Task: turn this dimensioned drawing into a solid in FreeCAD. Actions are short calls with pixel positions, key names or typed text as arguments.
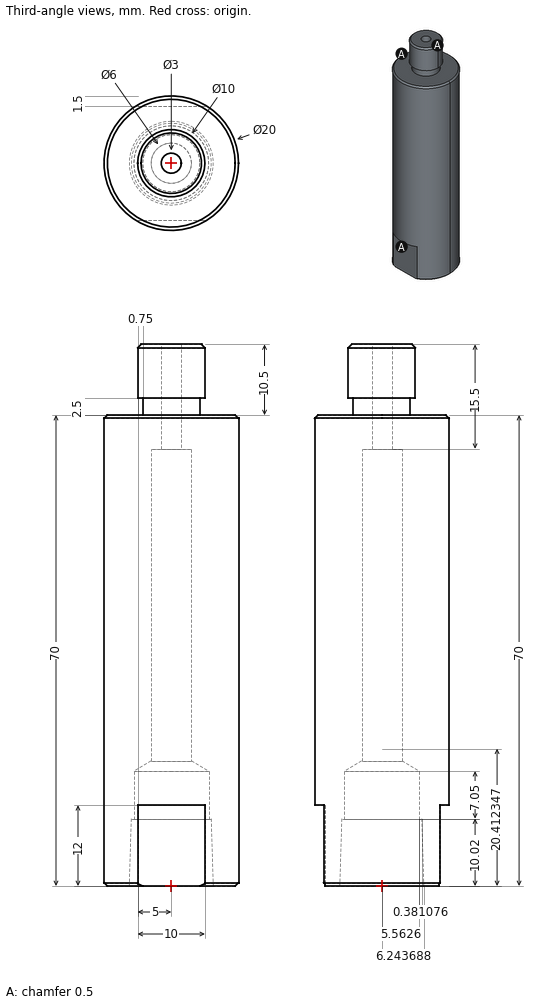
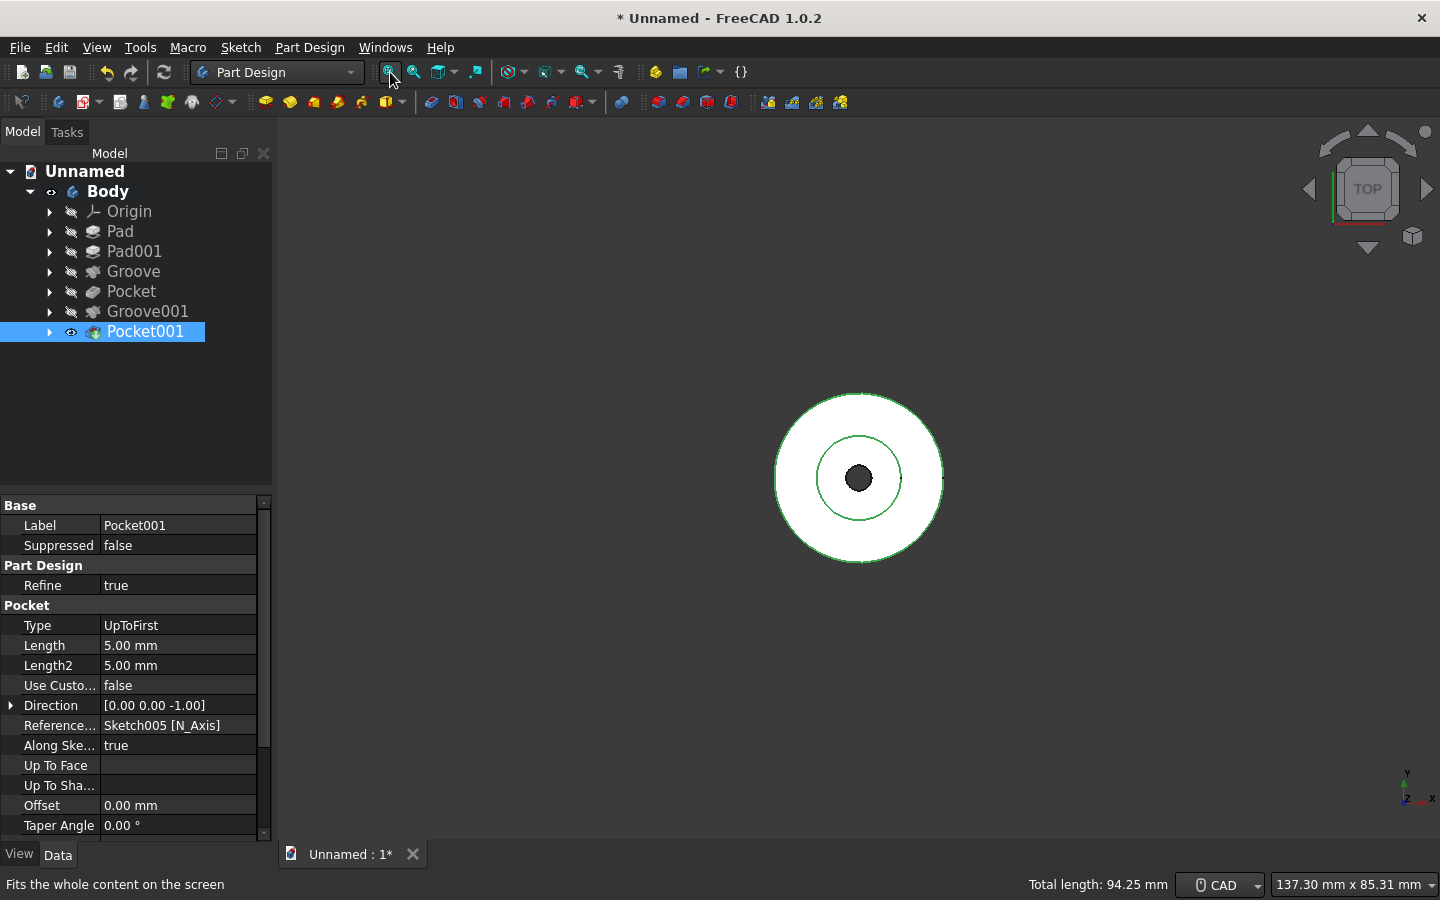
key(1)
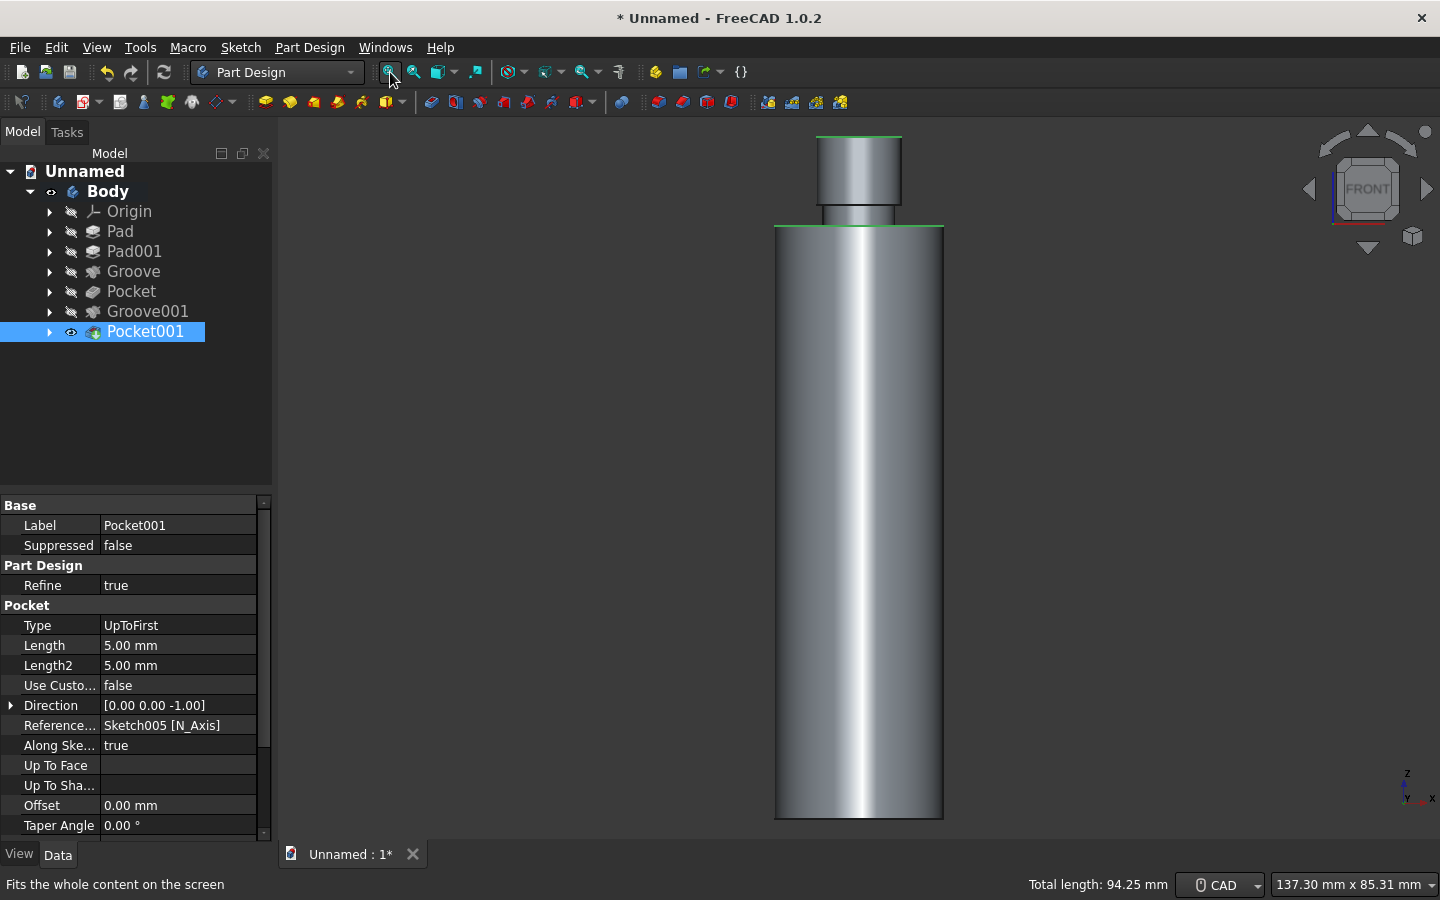
key(3)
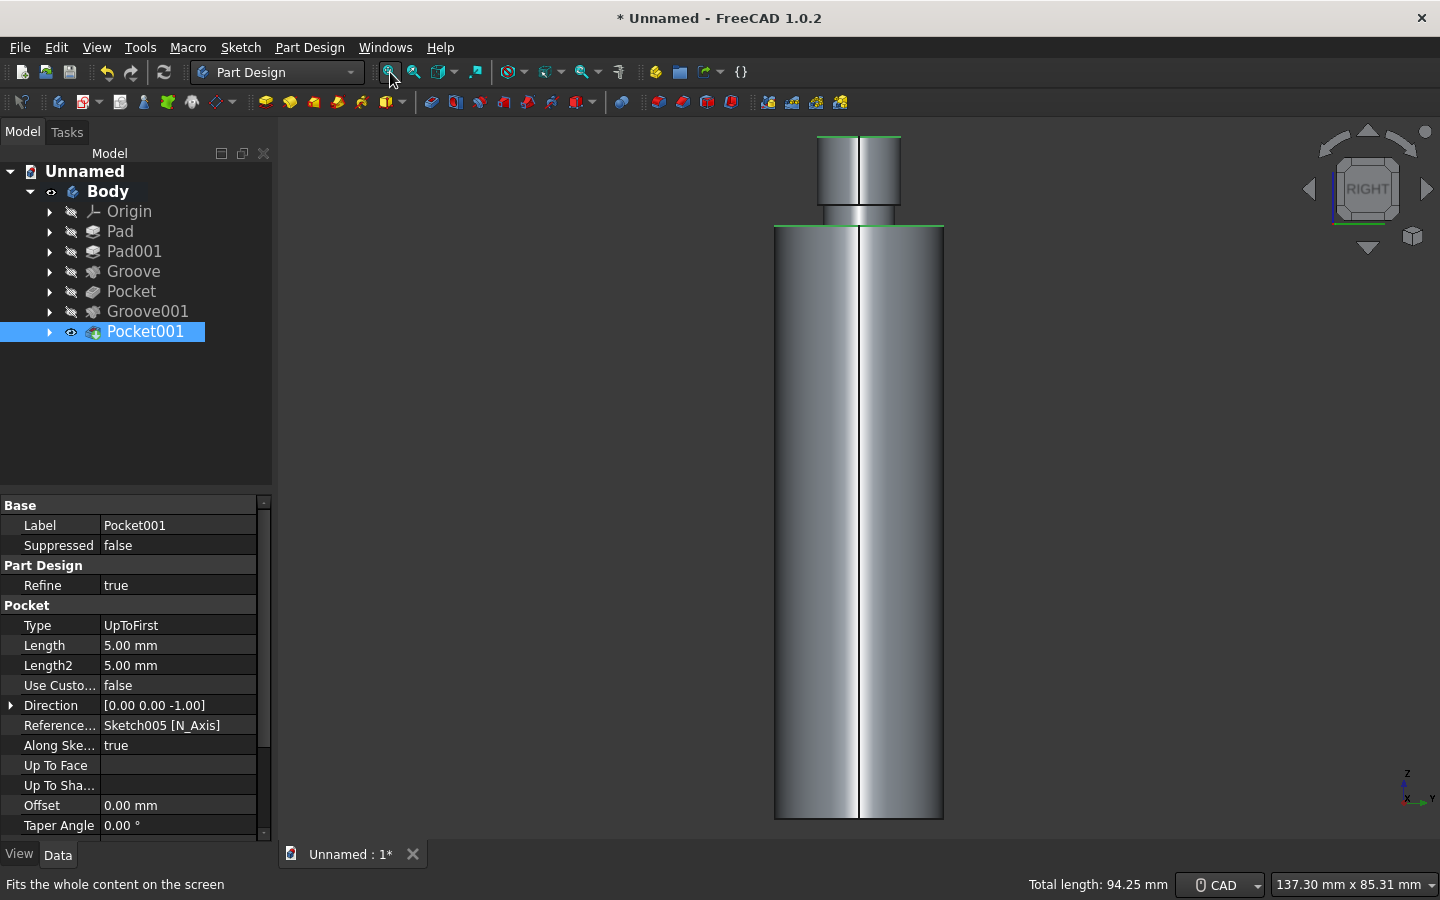
key(5)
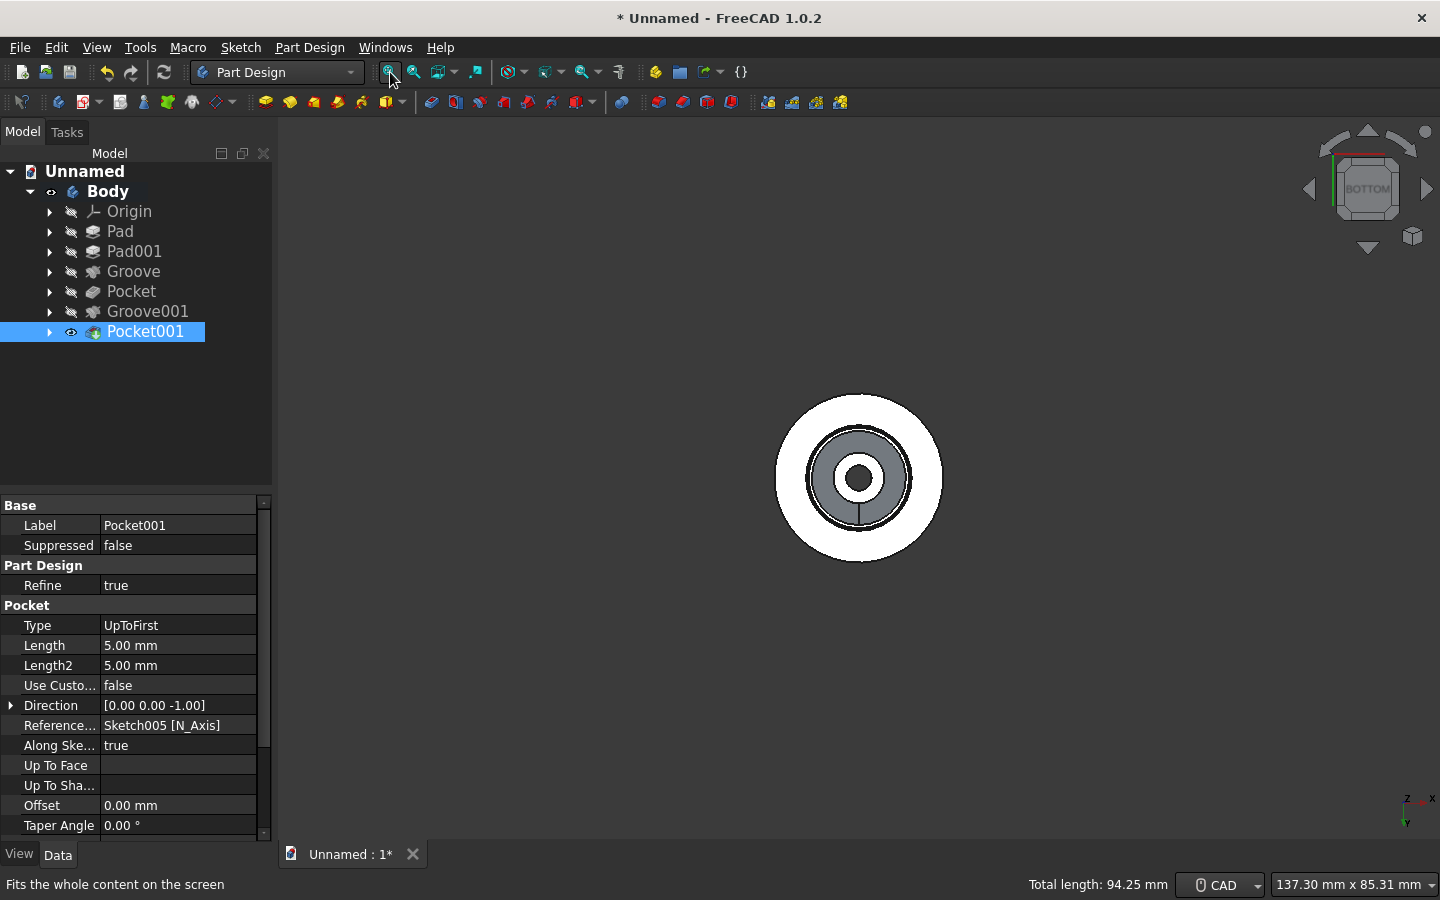
click(390, 72)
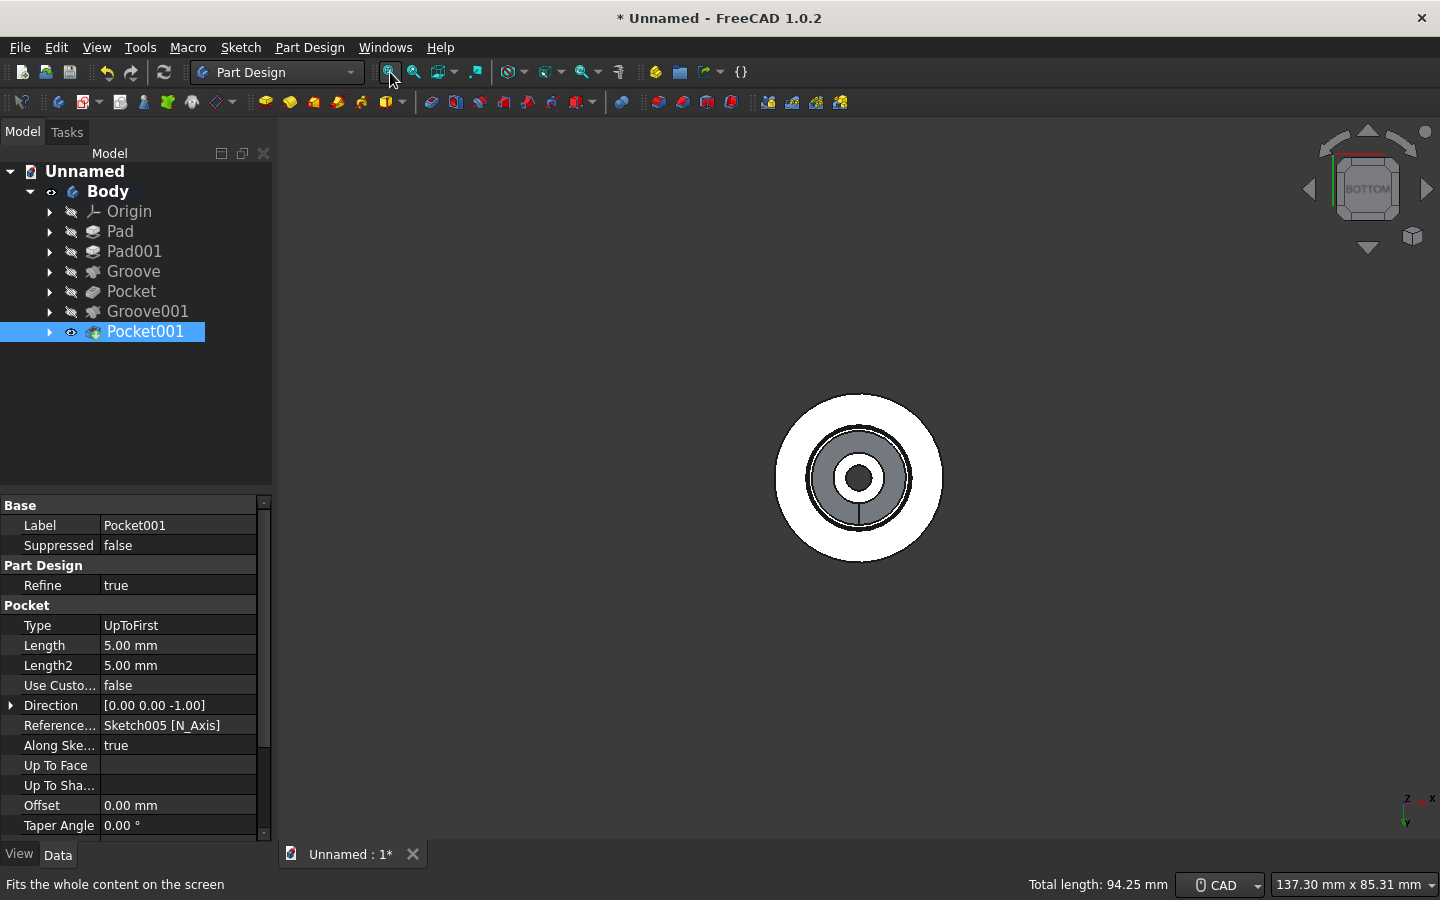
click(774, 477, ctrl)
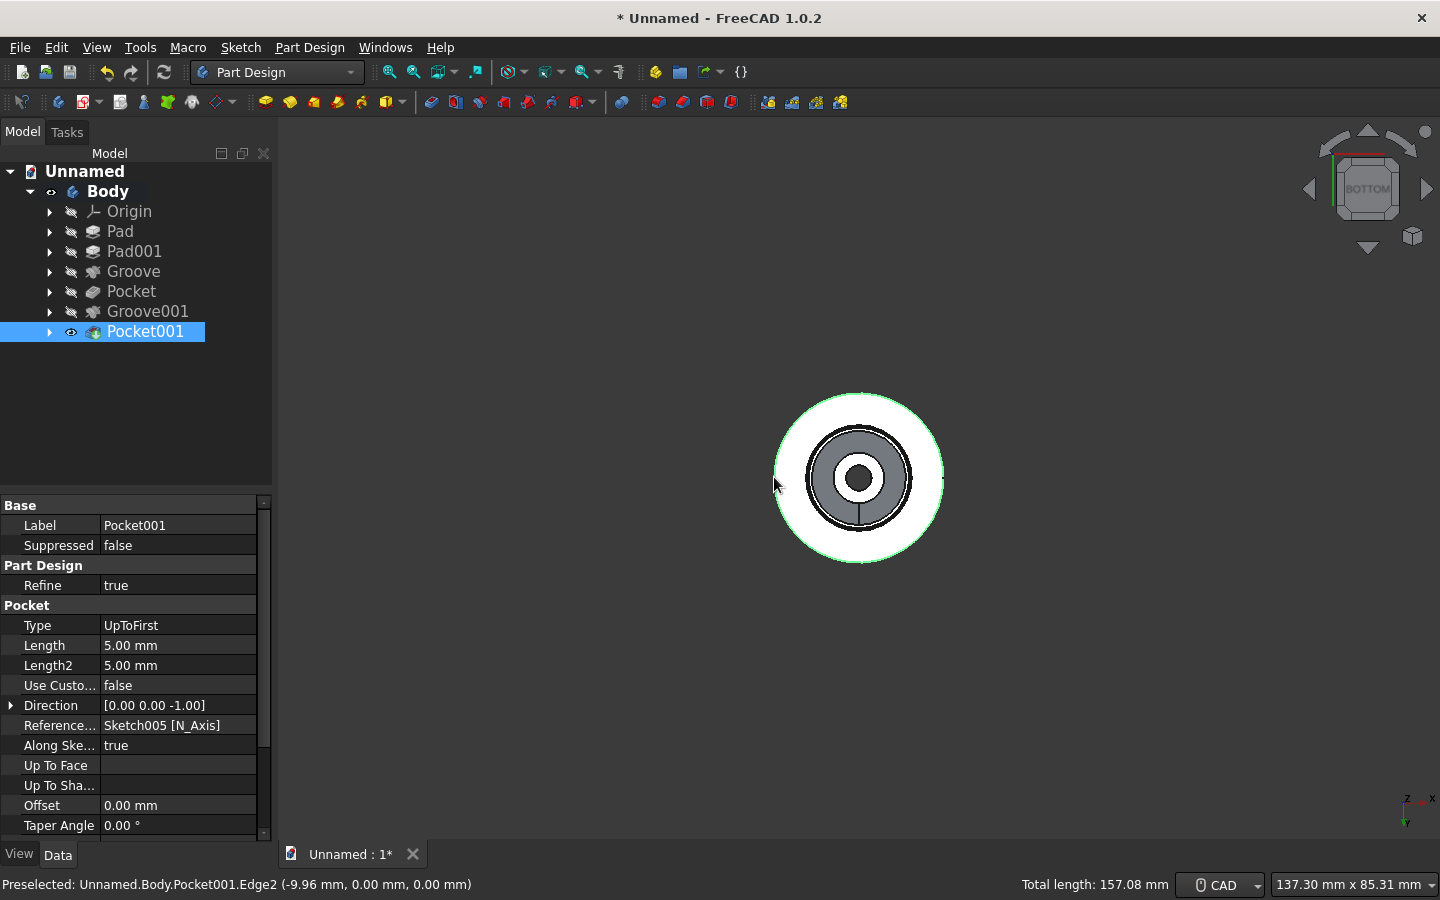
click(684, 102)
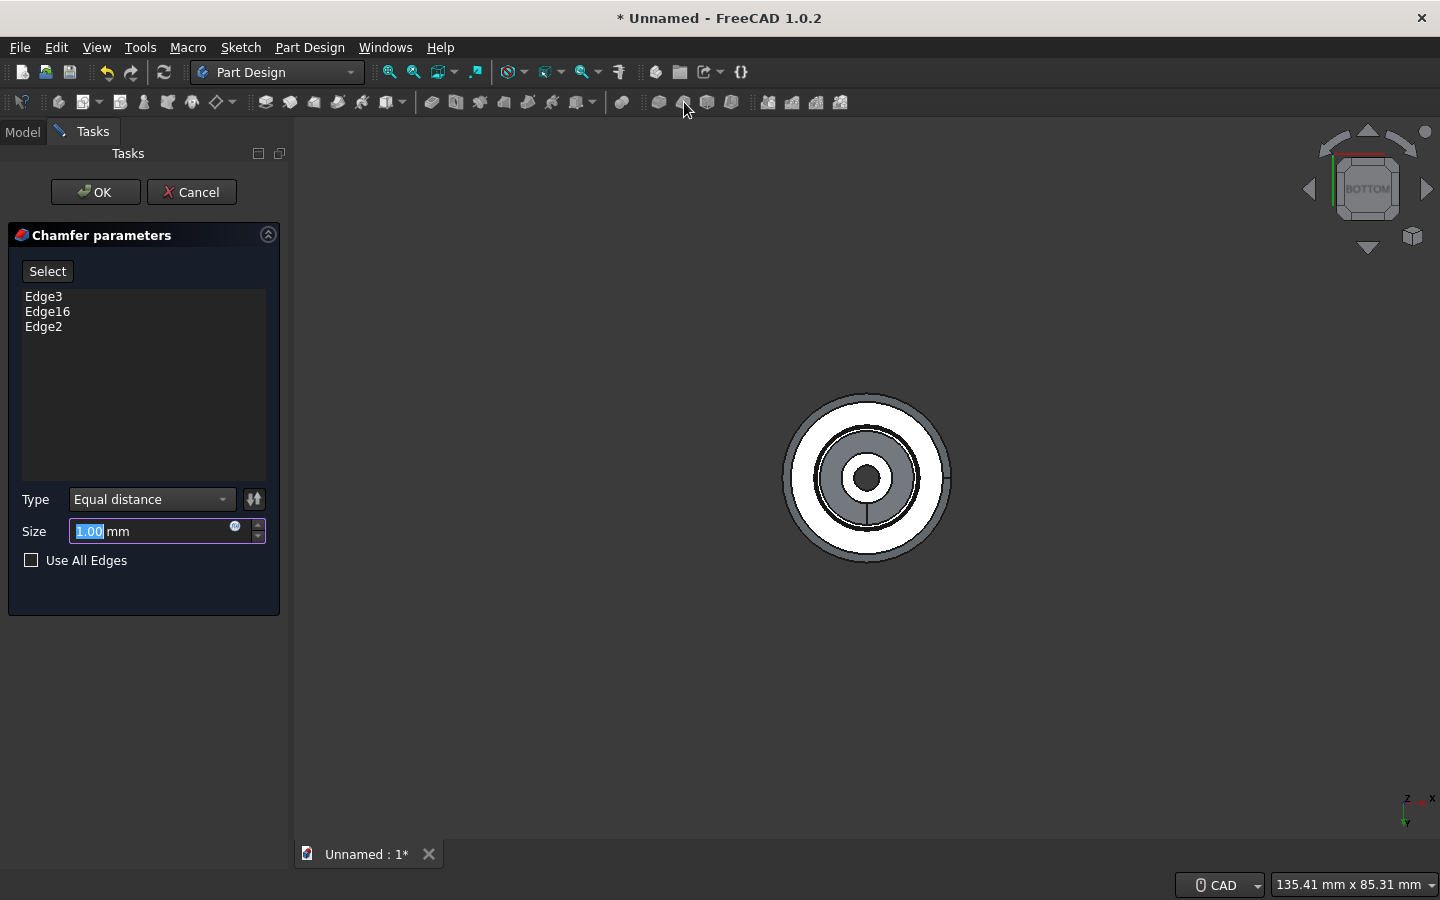
text(0.5)
key(Tab)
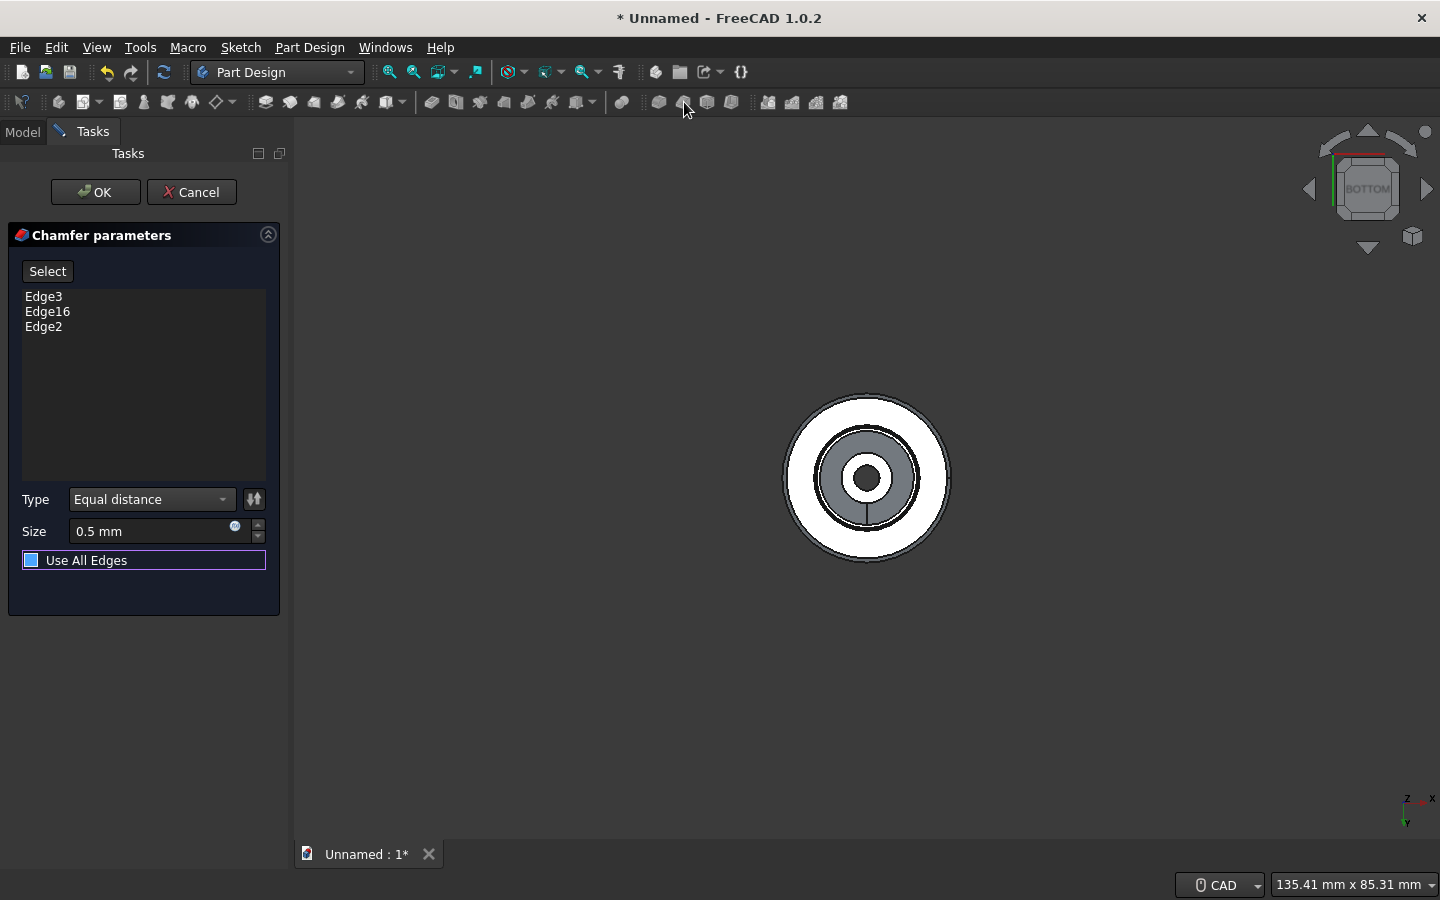
click(96, 192)